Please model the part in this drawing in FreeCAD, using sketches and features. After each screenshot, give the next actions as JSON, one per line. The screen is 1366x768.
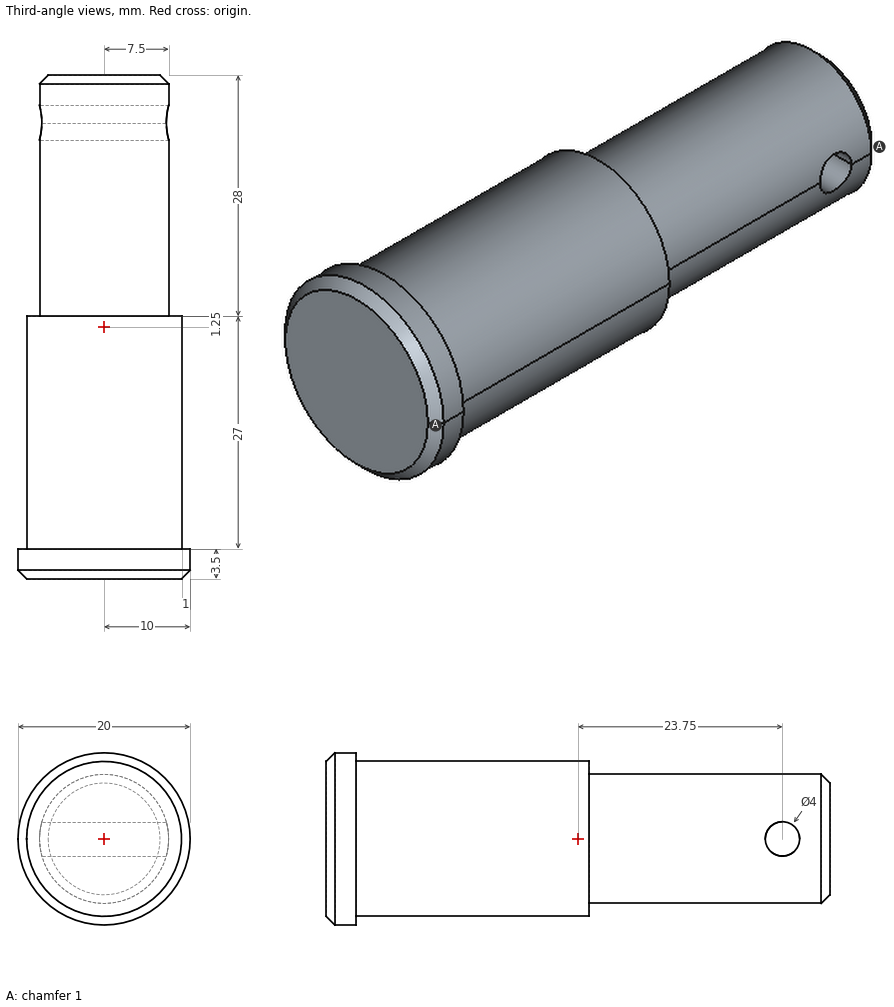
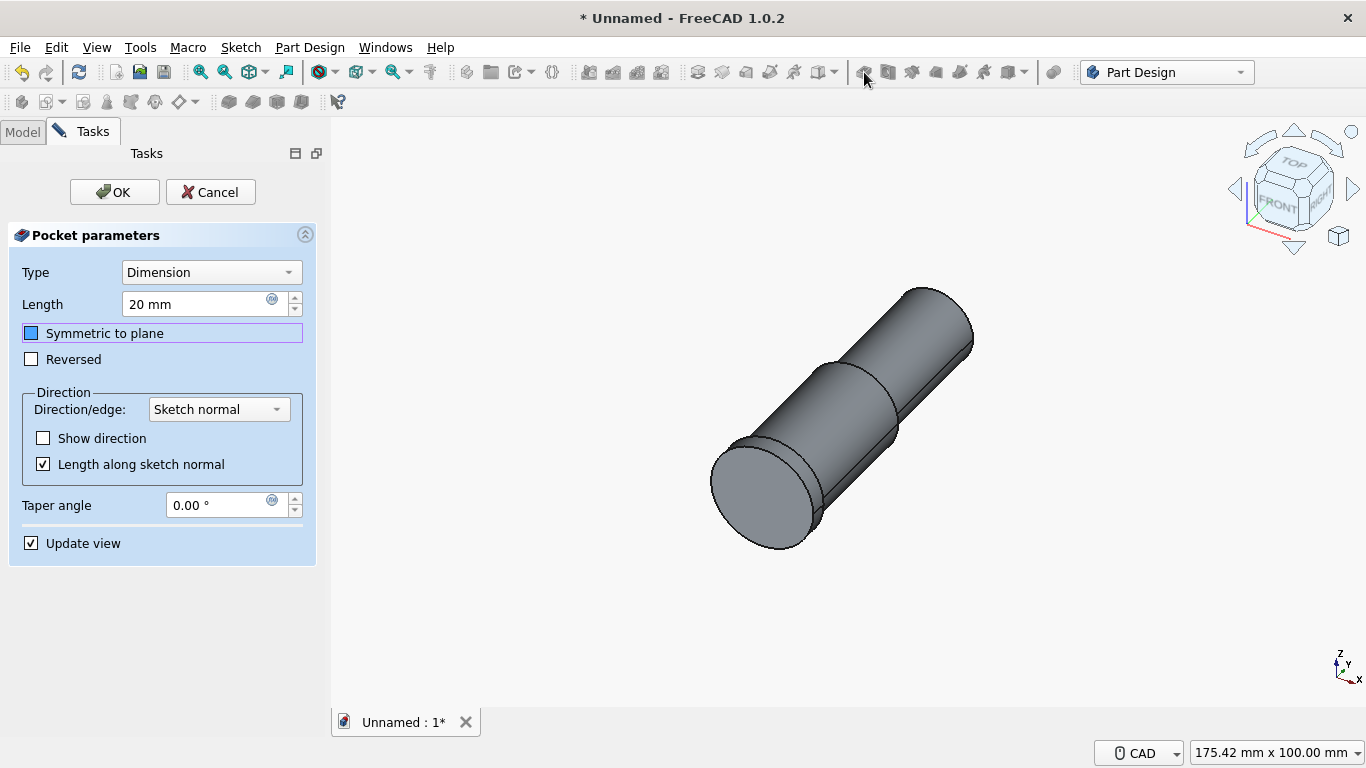
{"action": "left_click", "coordinate": [30, 333]}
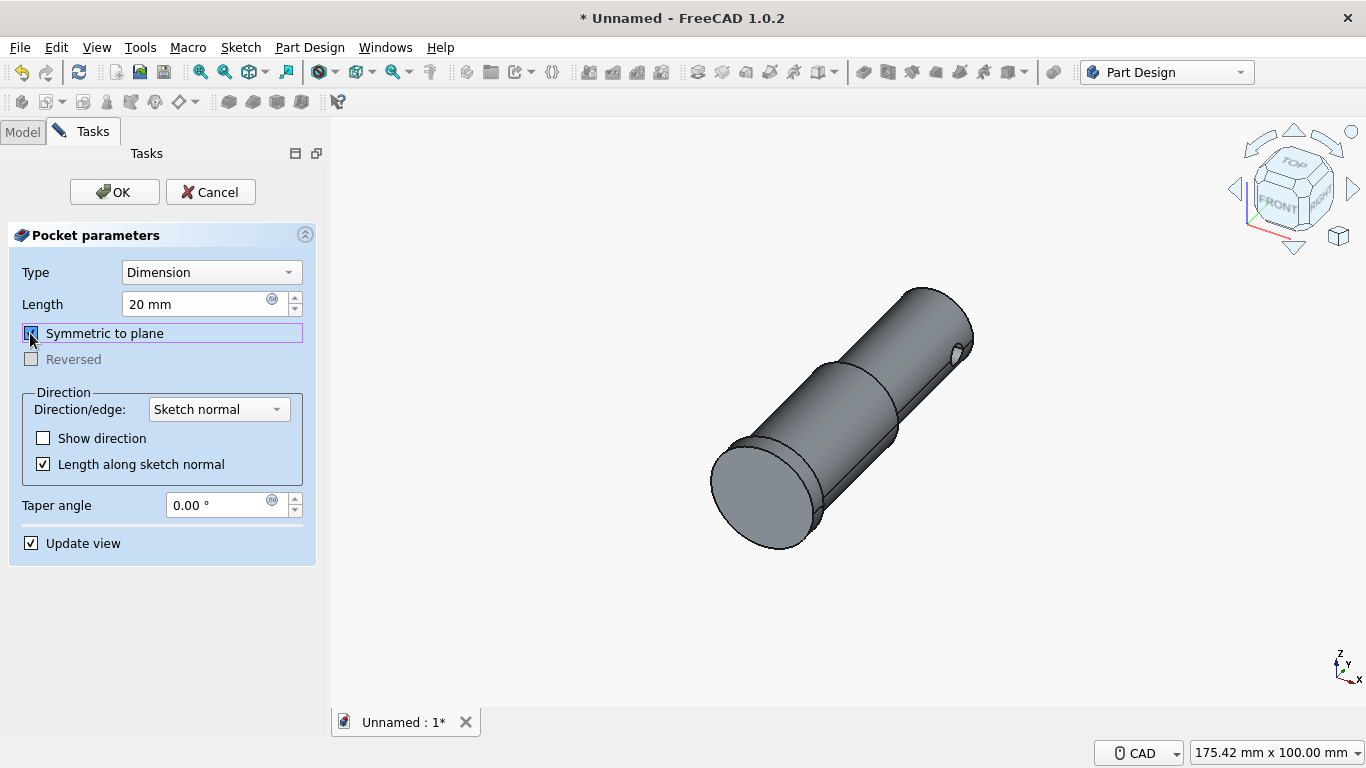
{"action": "left_click", "coordinate": [115, 192]}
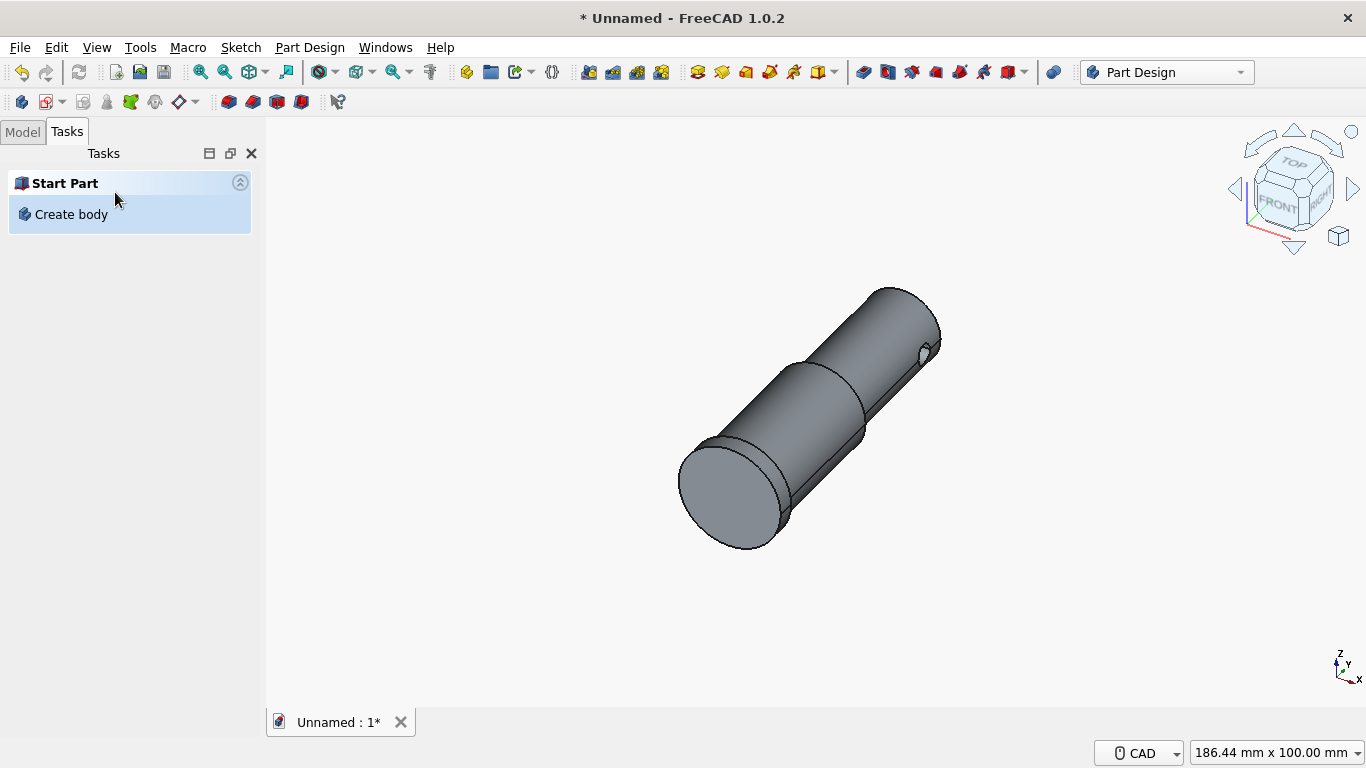
{"action": "left_click", "coordinate": [688, 455]}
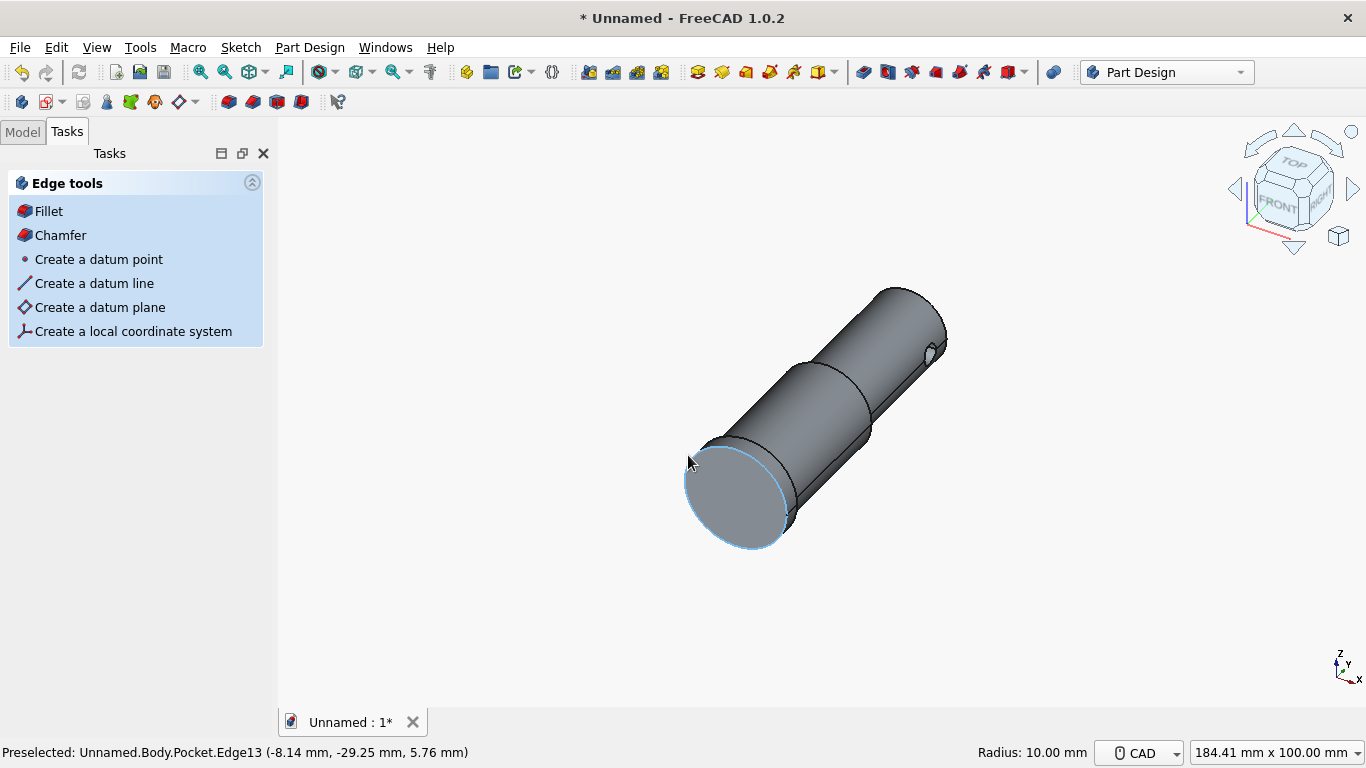
{"action": "key", "text": "0"}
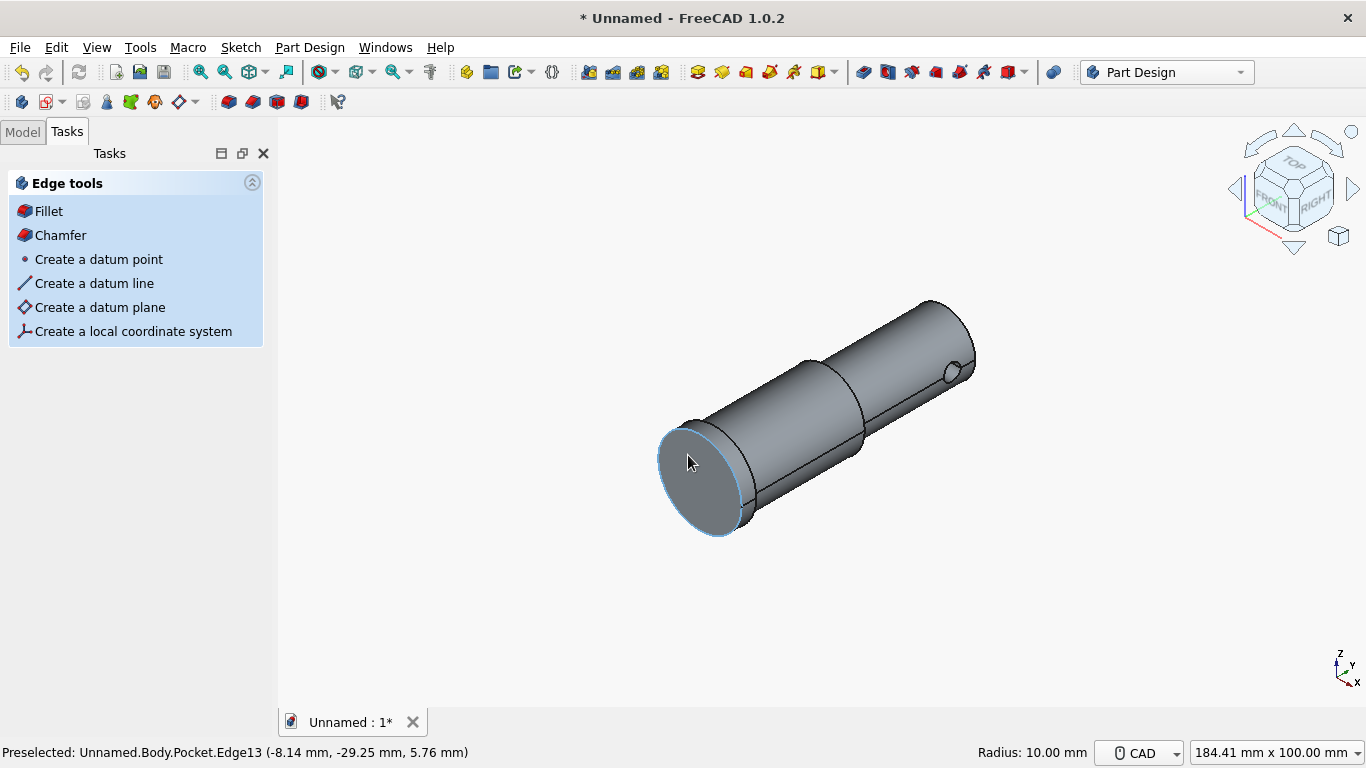
{"action": "key", "text": "2"}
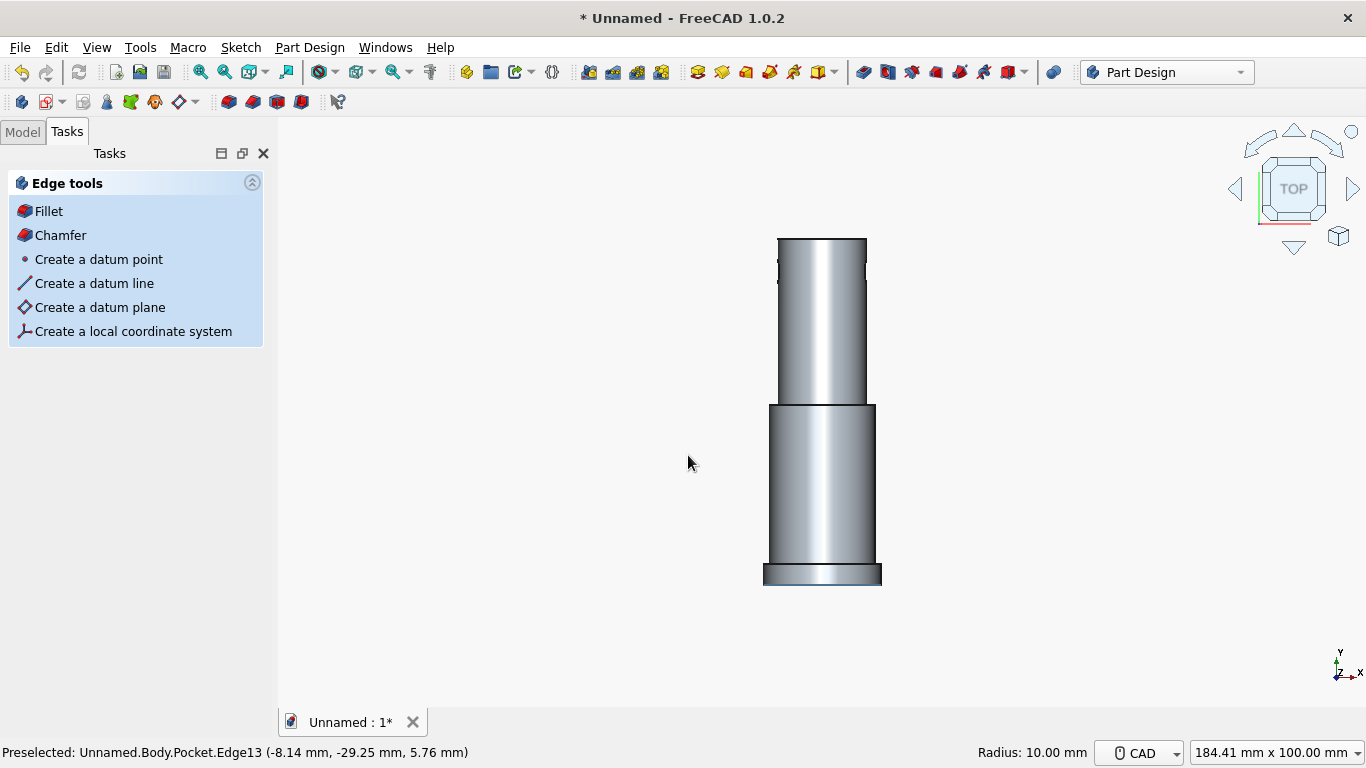
{"action": "left_click", "coordinate": [786, 238], "text": "ctrl"}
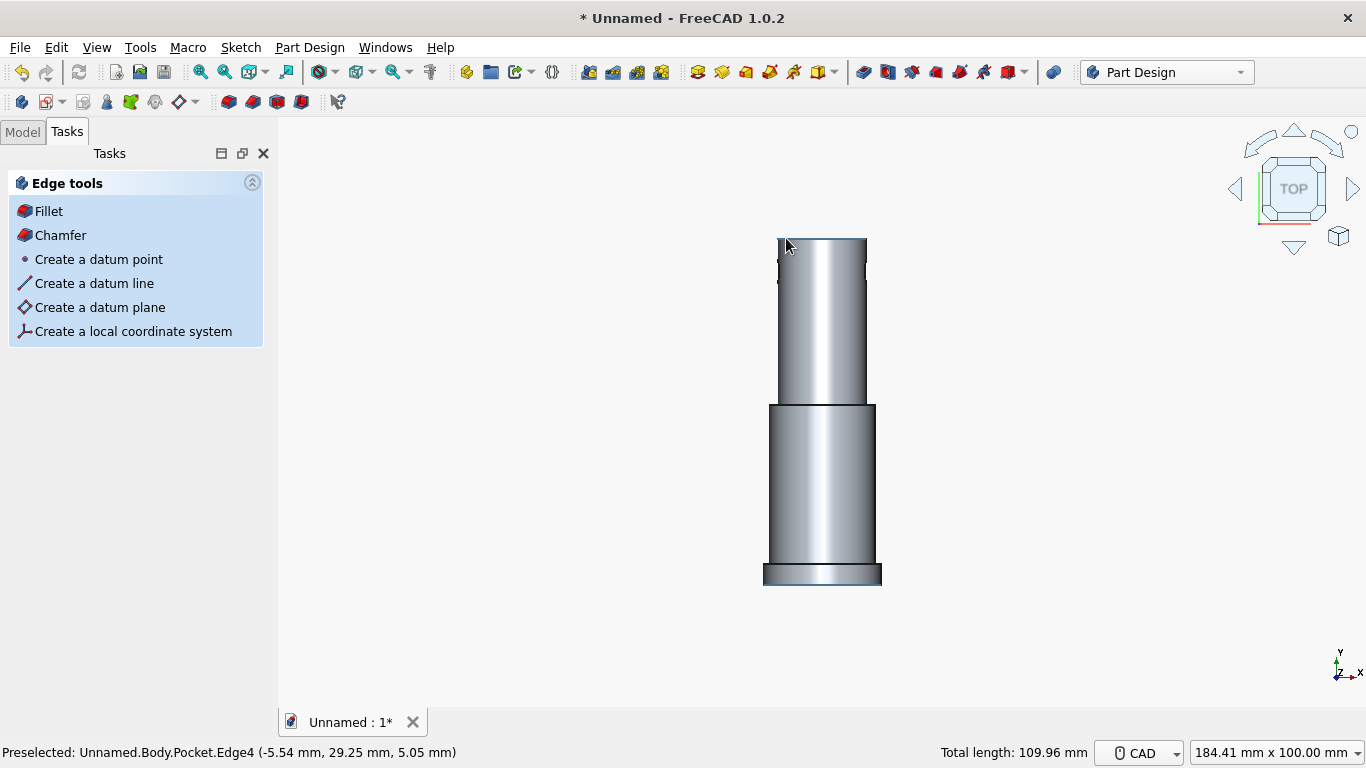
{"action": "left_click", "coordinate": [254, 102]}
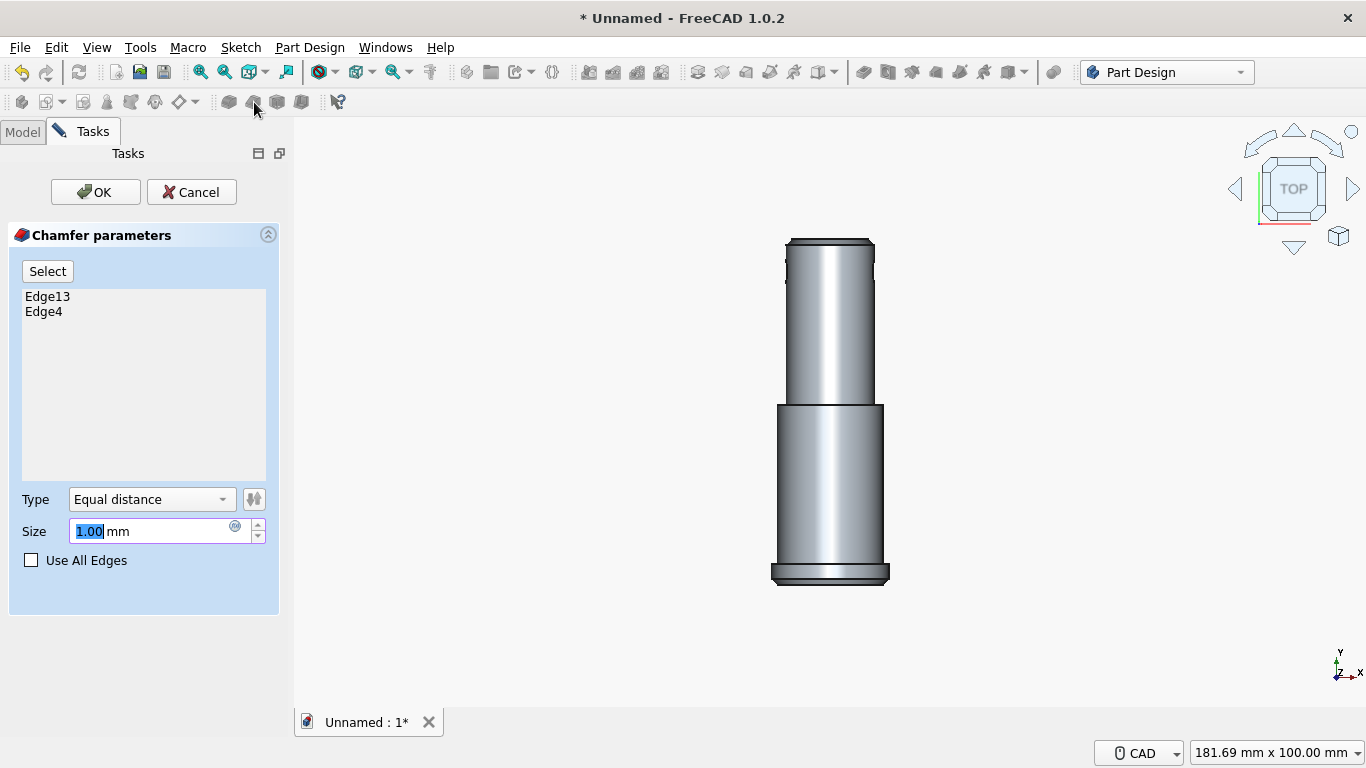
{"action": "type", "text": "1"}
{"action": "key", "text": "Tab"}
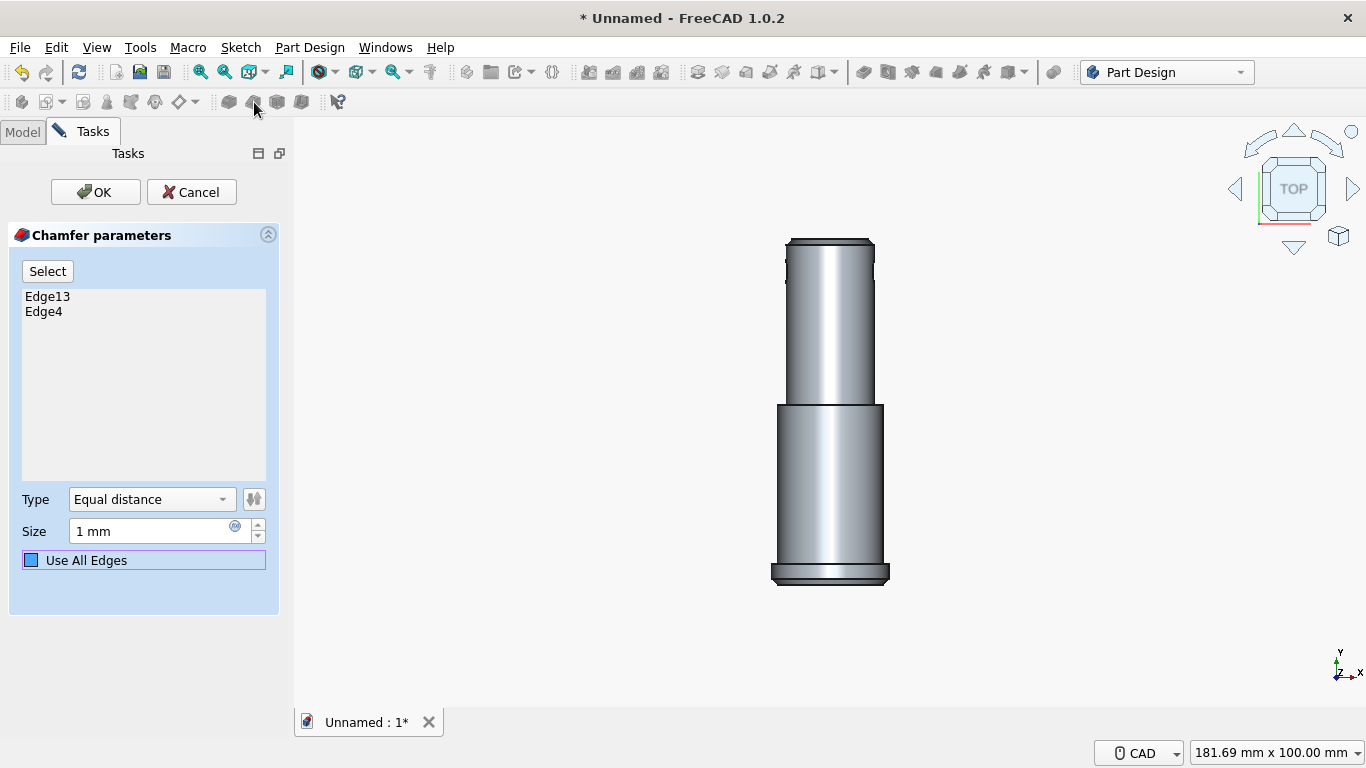
{"action": "left_click", "coordinate": [96, 192]}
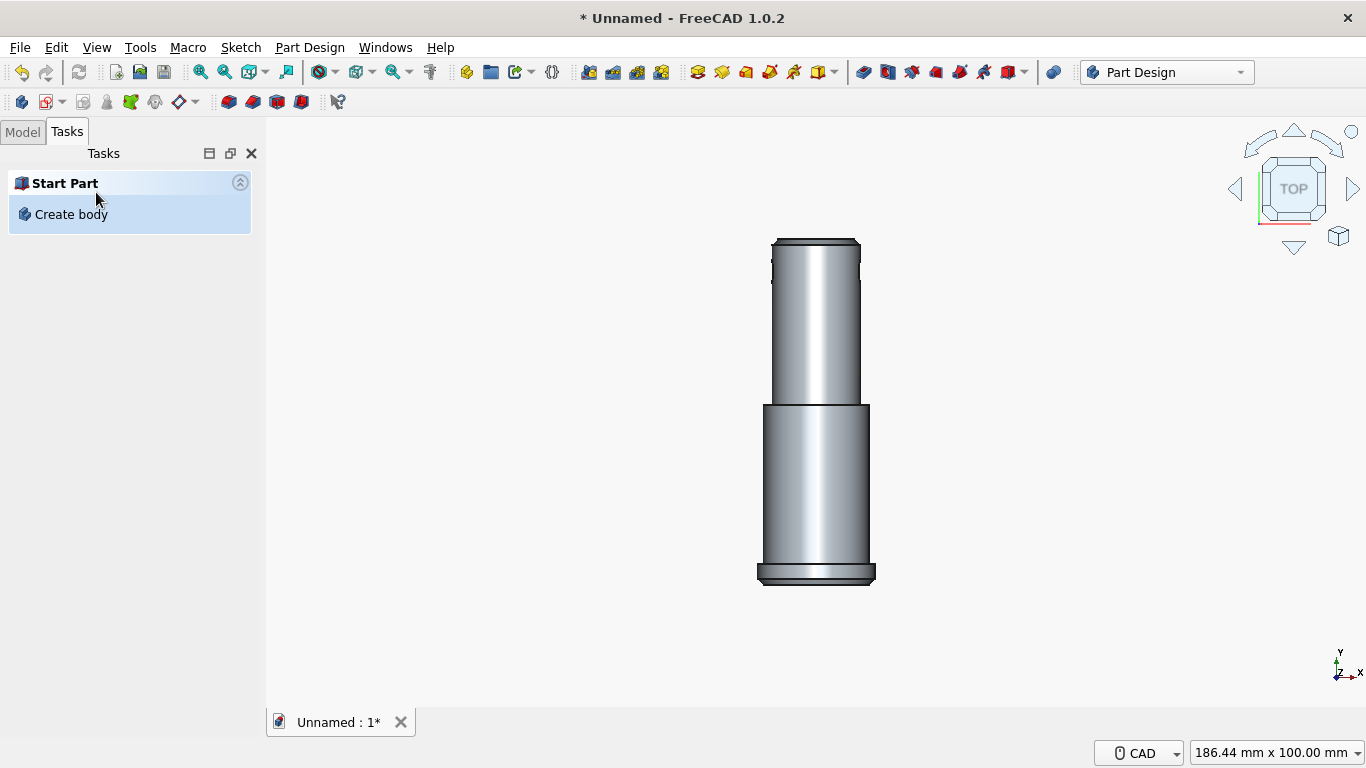
{"action": "key", "text": "0"}